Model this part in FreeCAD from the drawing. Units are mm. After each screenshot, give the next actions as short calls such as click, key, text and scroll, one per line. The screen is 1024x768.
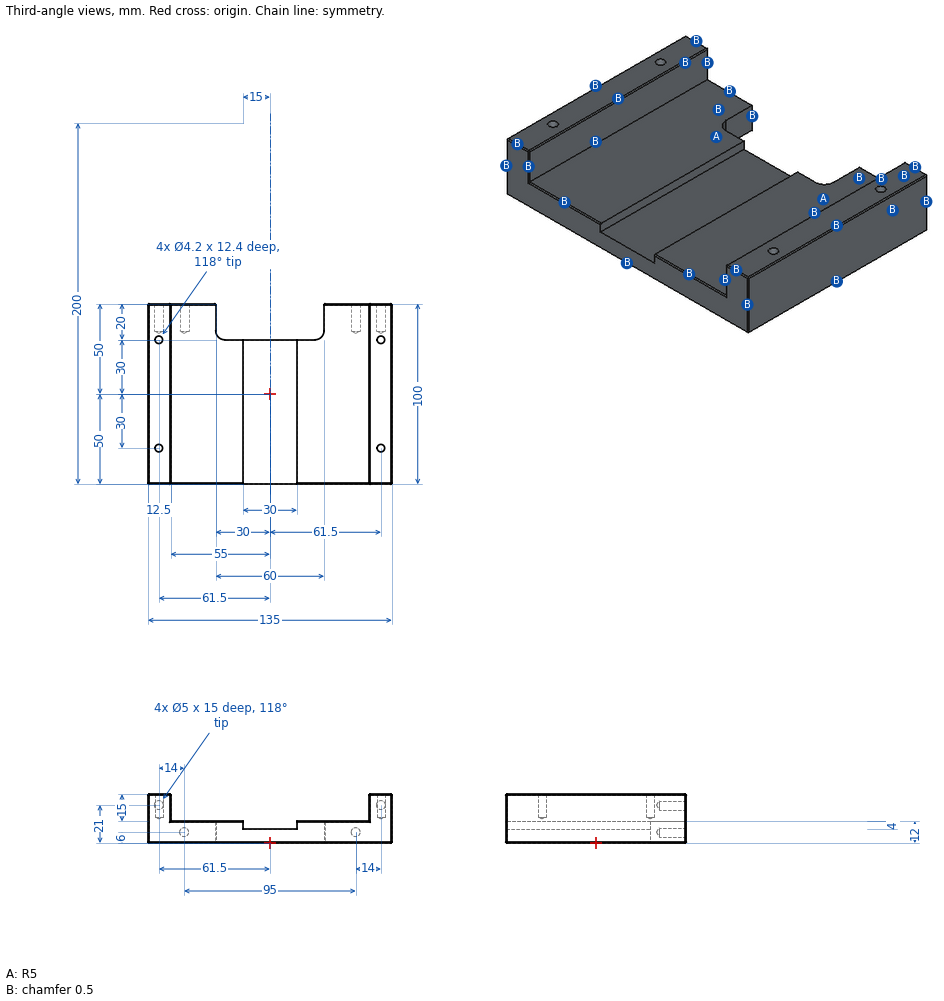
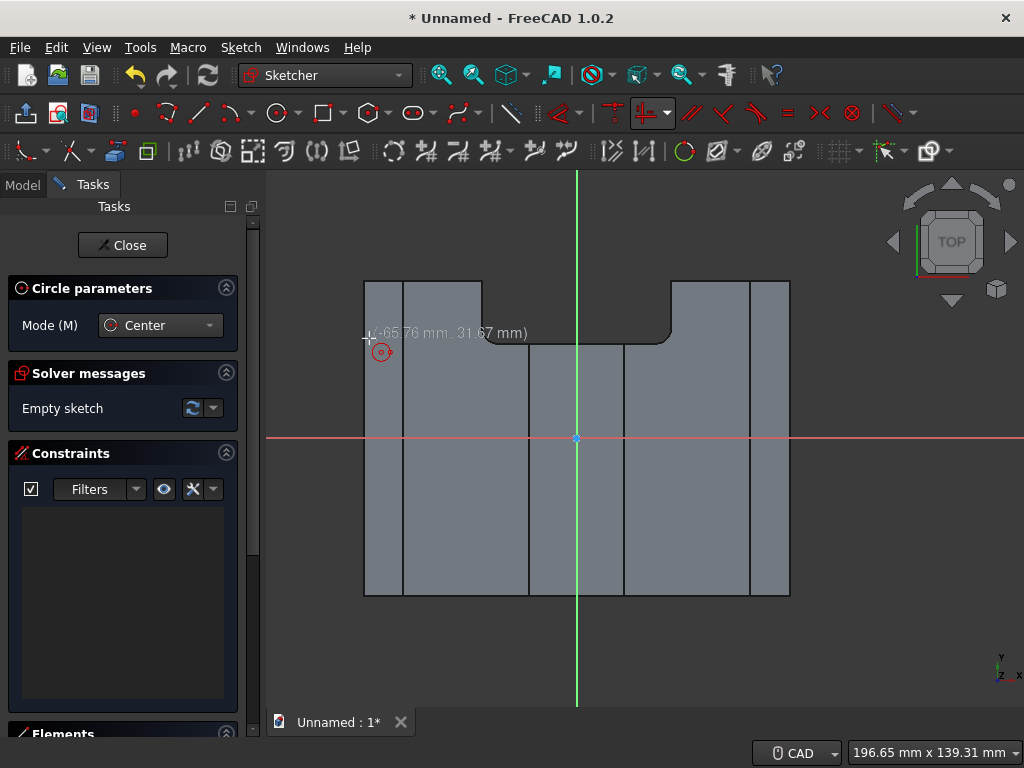
click(383, 344)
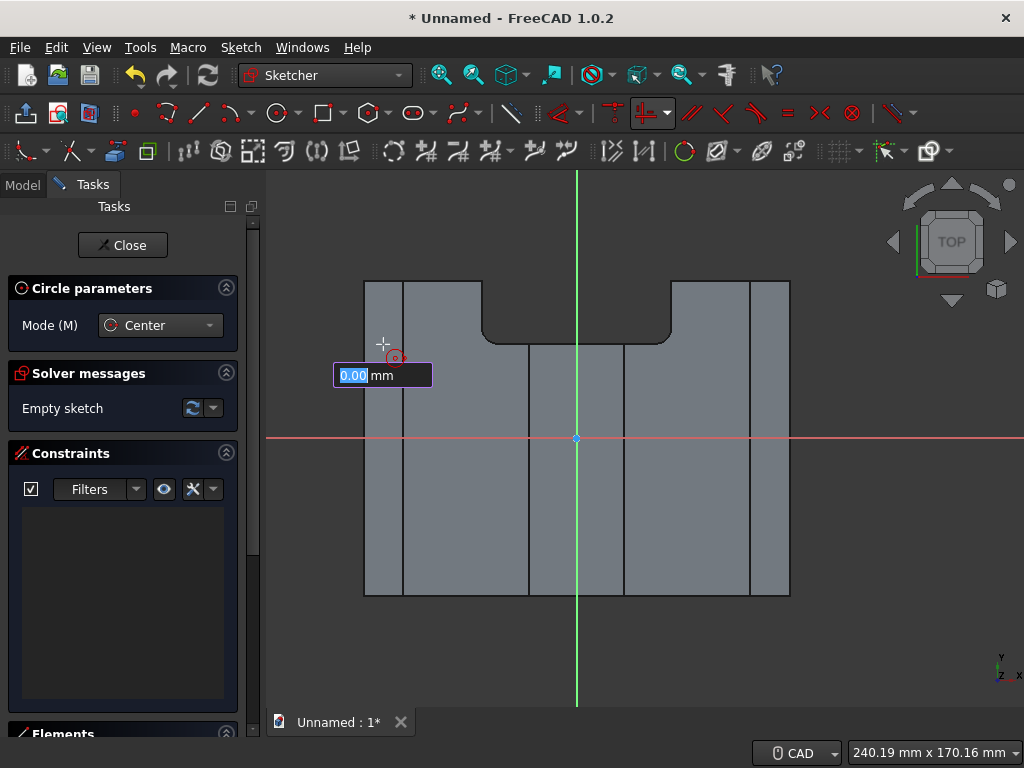
scroll(387, 339, up, 5)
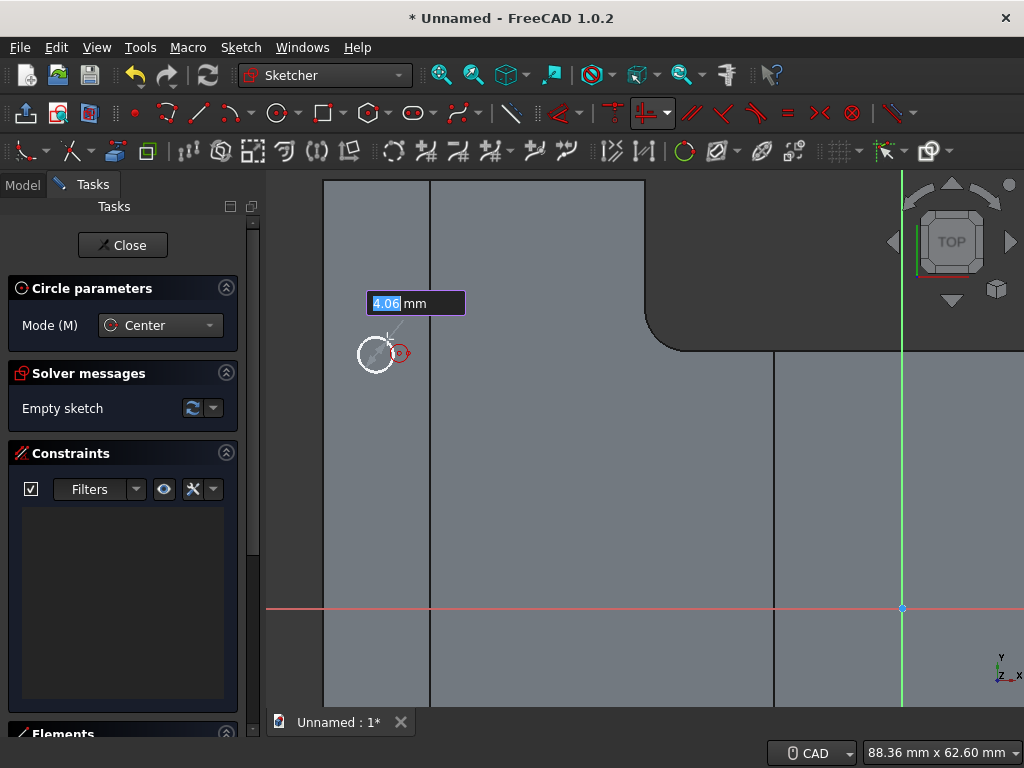
click(387, 339)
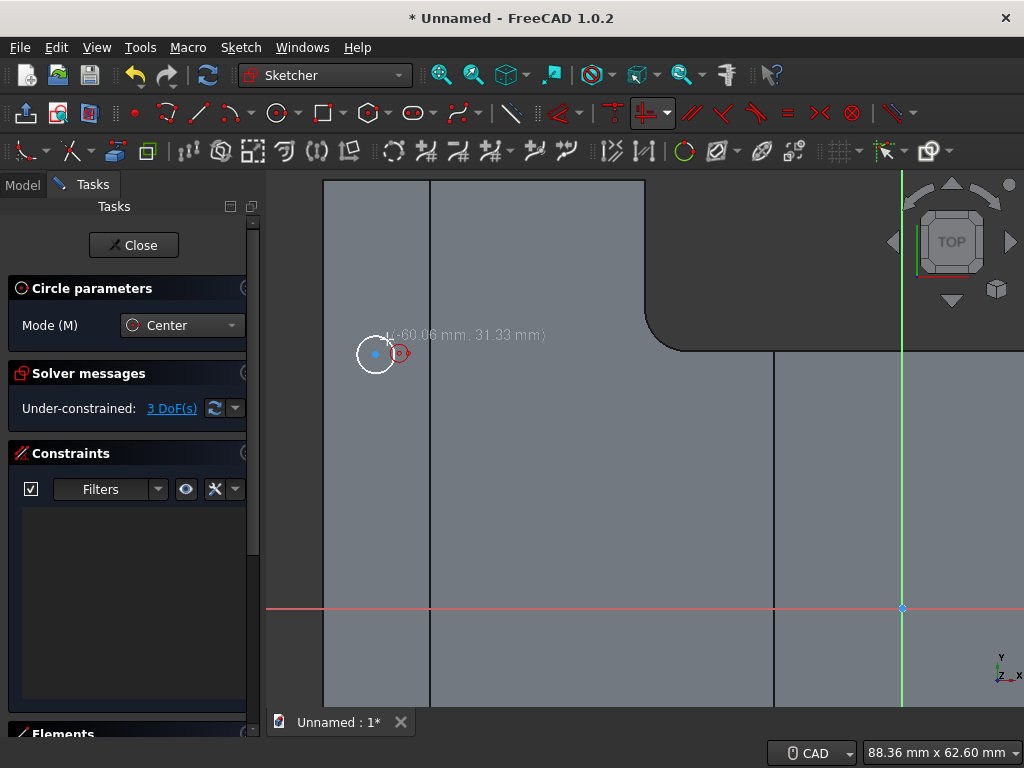
scroll(387, 339, down, 5)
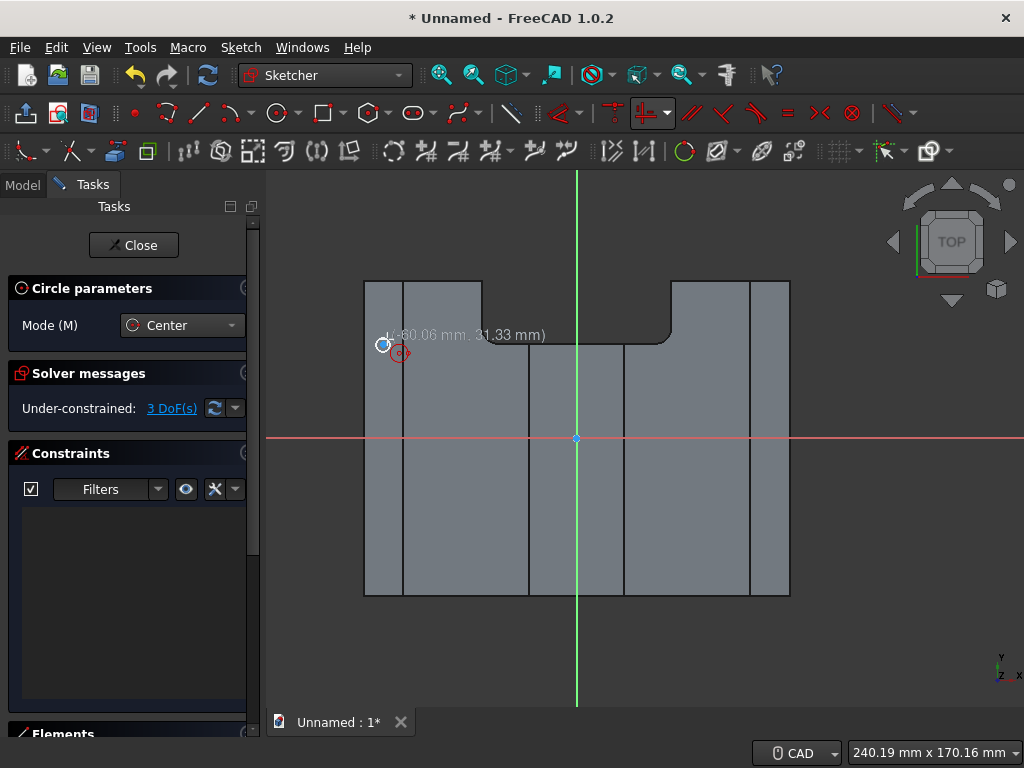
scroll(383, 533, up, 7)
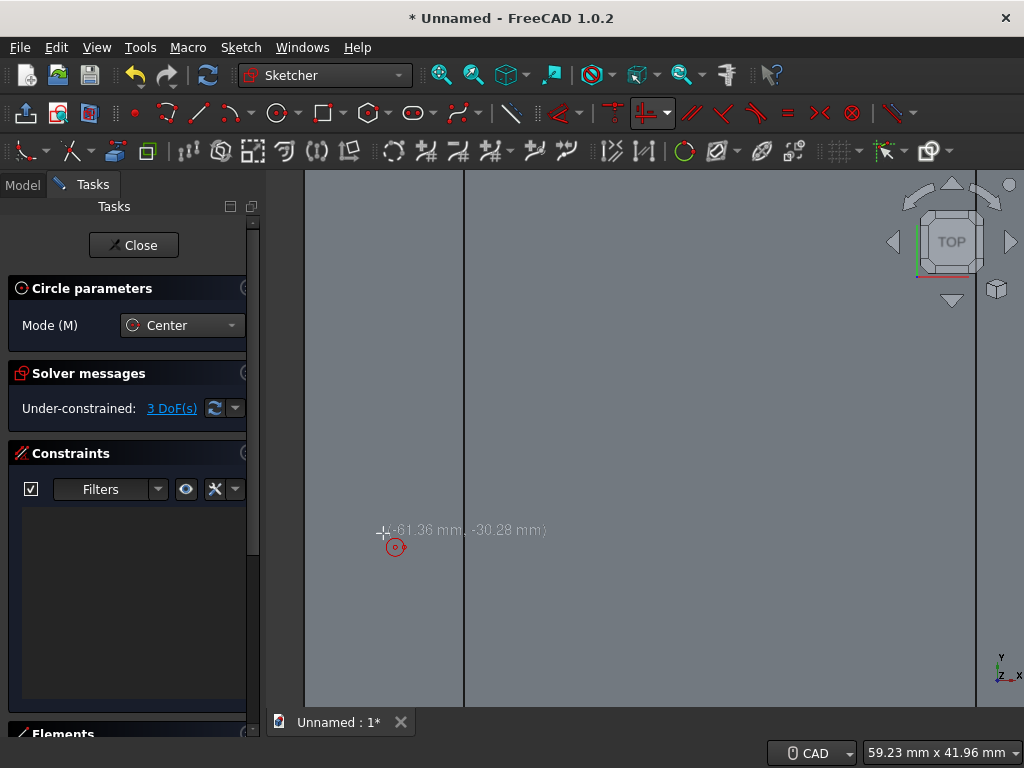
scroll(383, 534, down, 7)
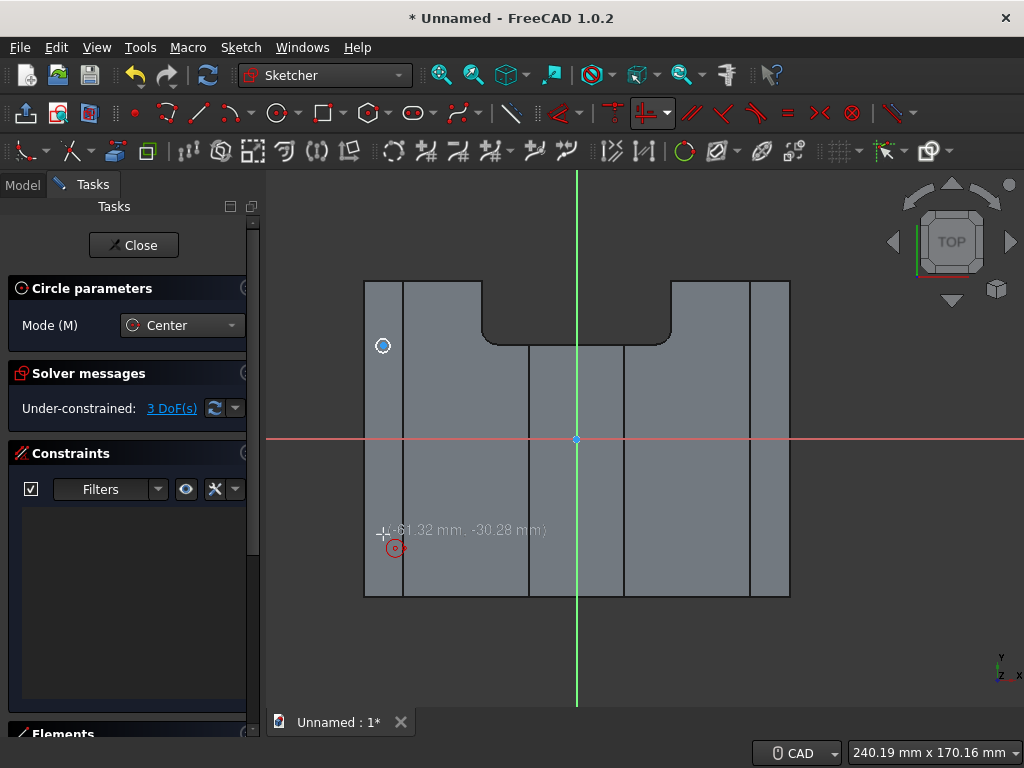
click(383, 534)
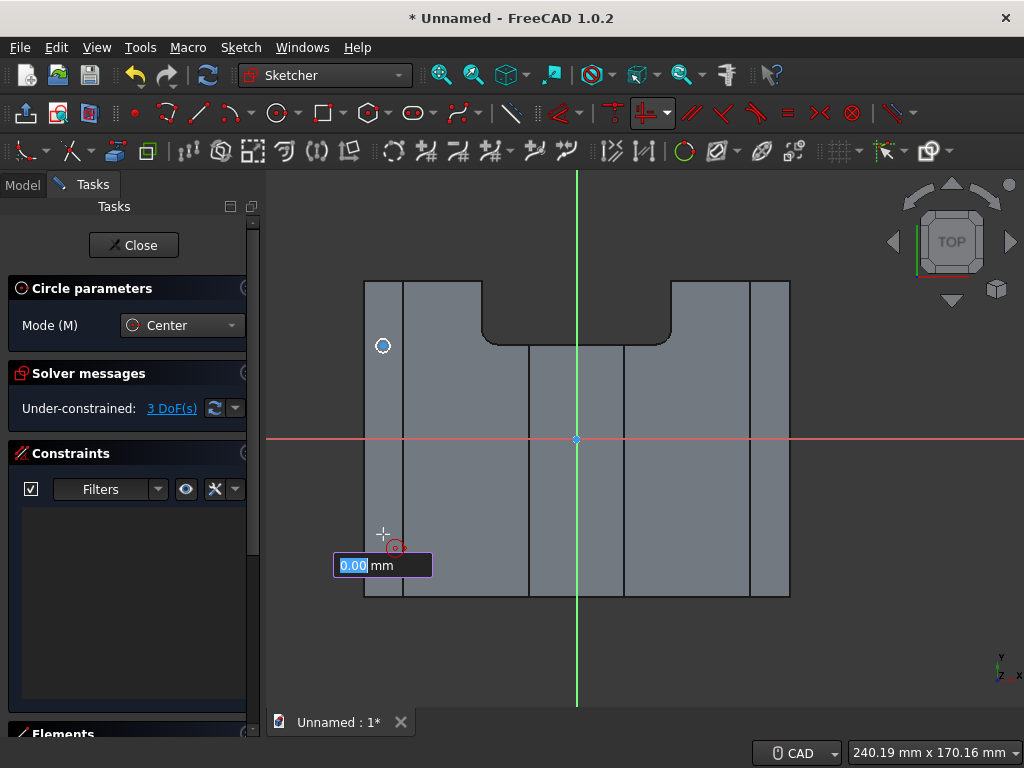
scroll(387, 529, up, 5)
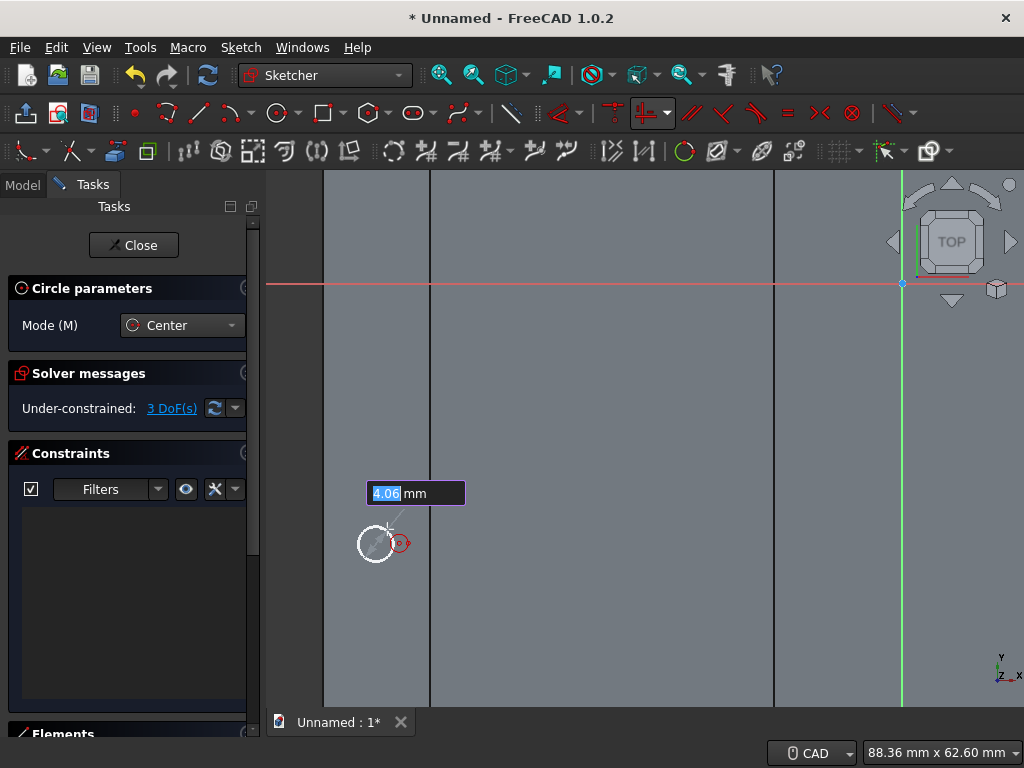
click(387, 528)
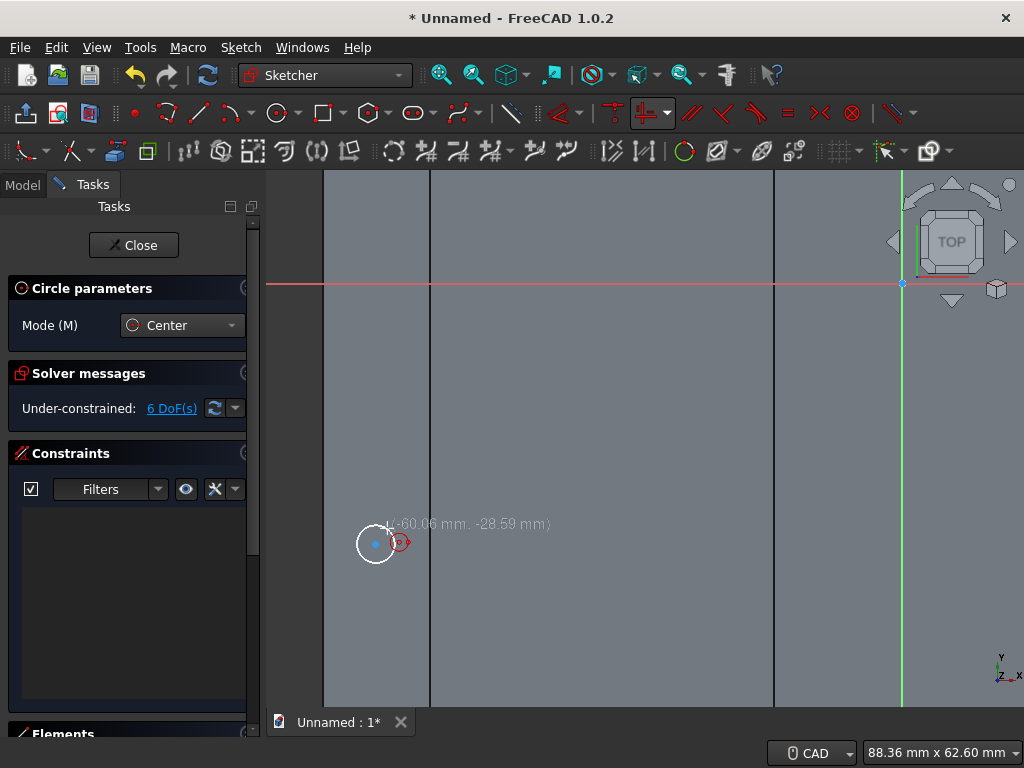
scroll(387, 529, down, 5)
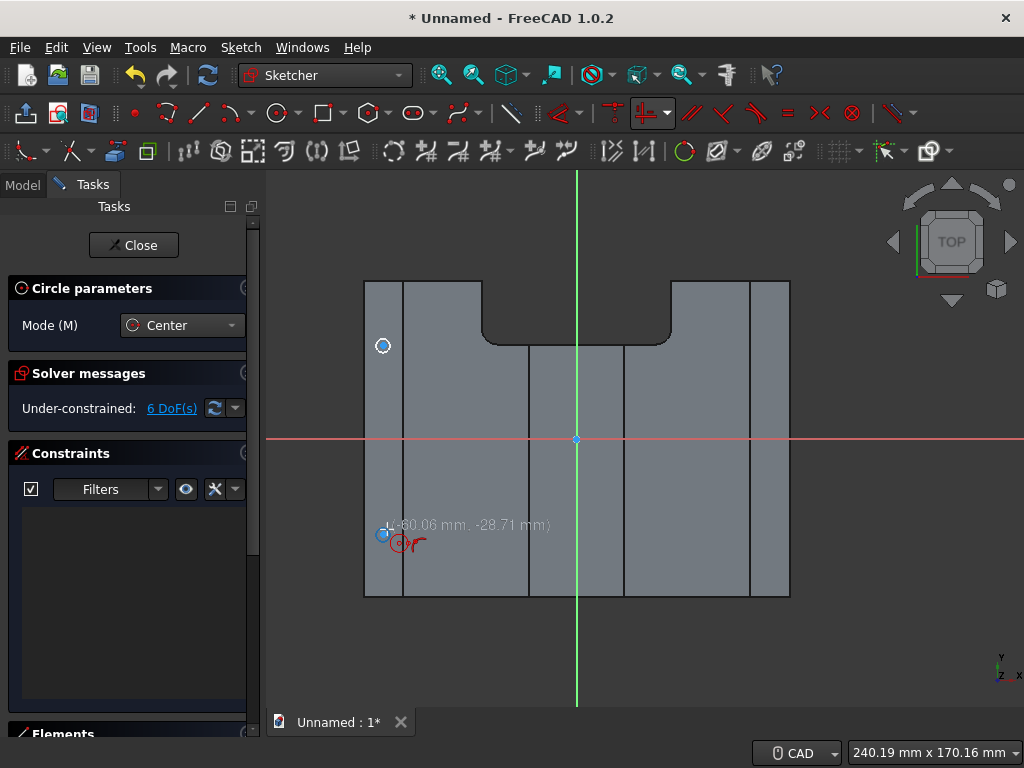
scroll(771, 534, up, 7)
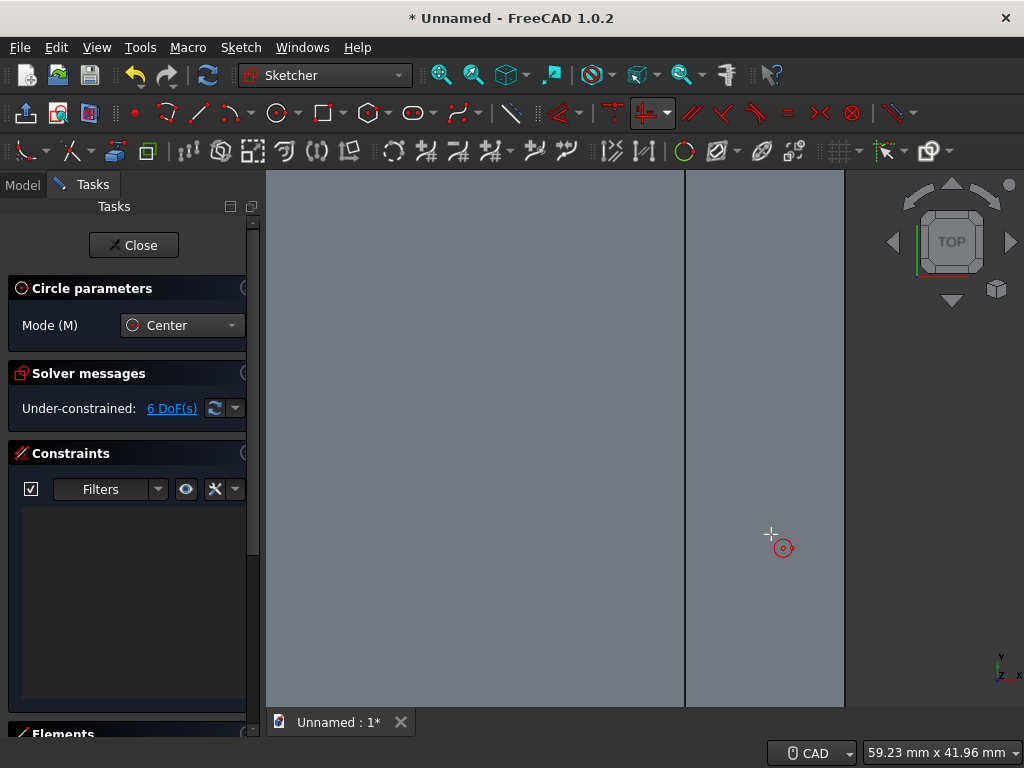
scroll(771, 534, down, 7)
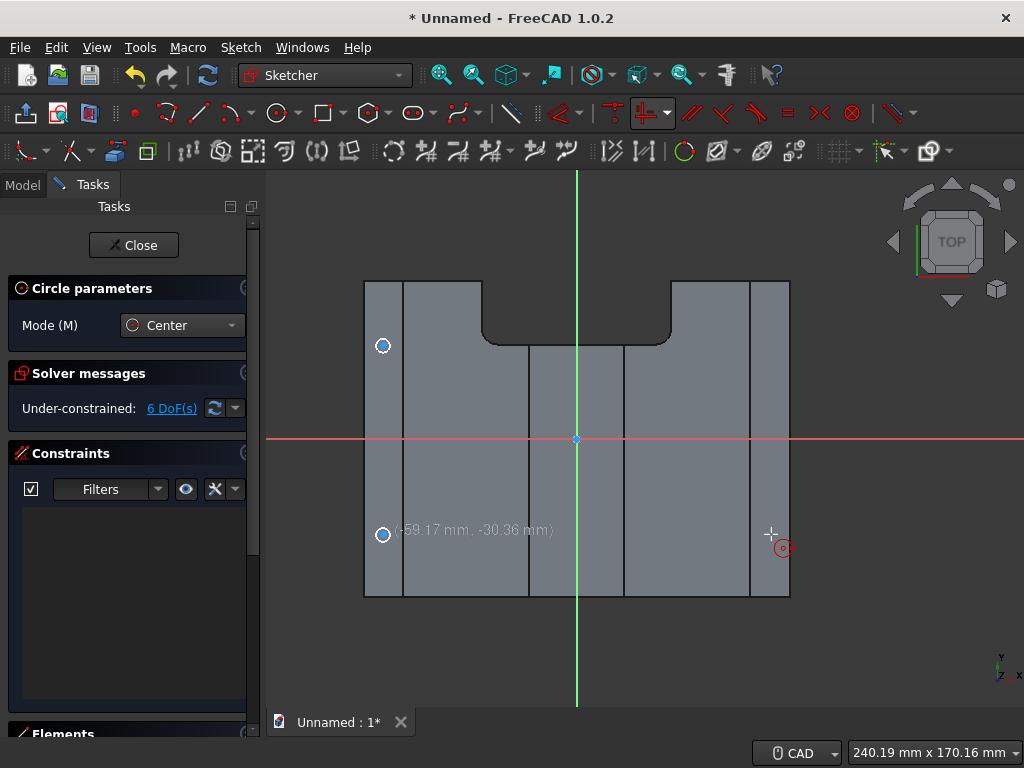
click(771, 534)